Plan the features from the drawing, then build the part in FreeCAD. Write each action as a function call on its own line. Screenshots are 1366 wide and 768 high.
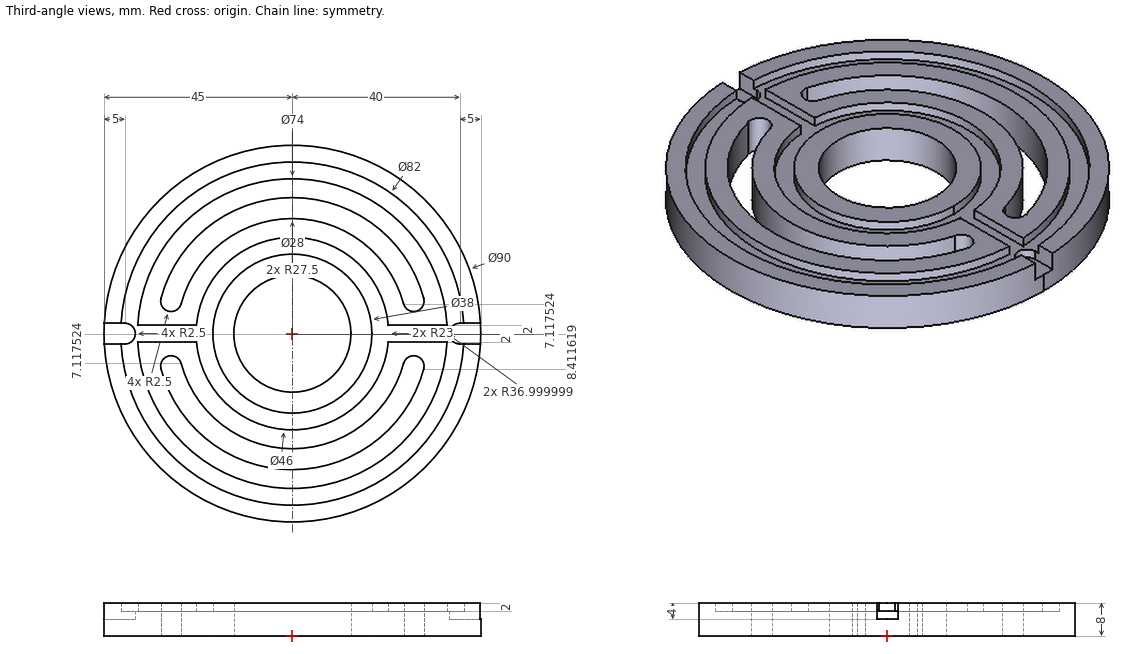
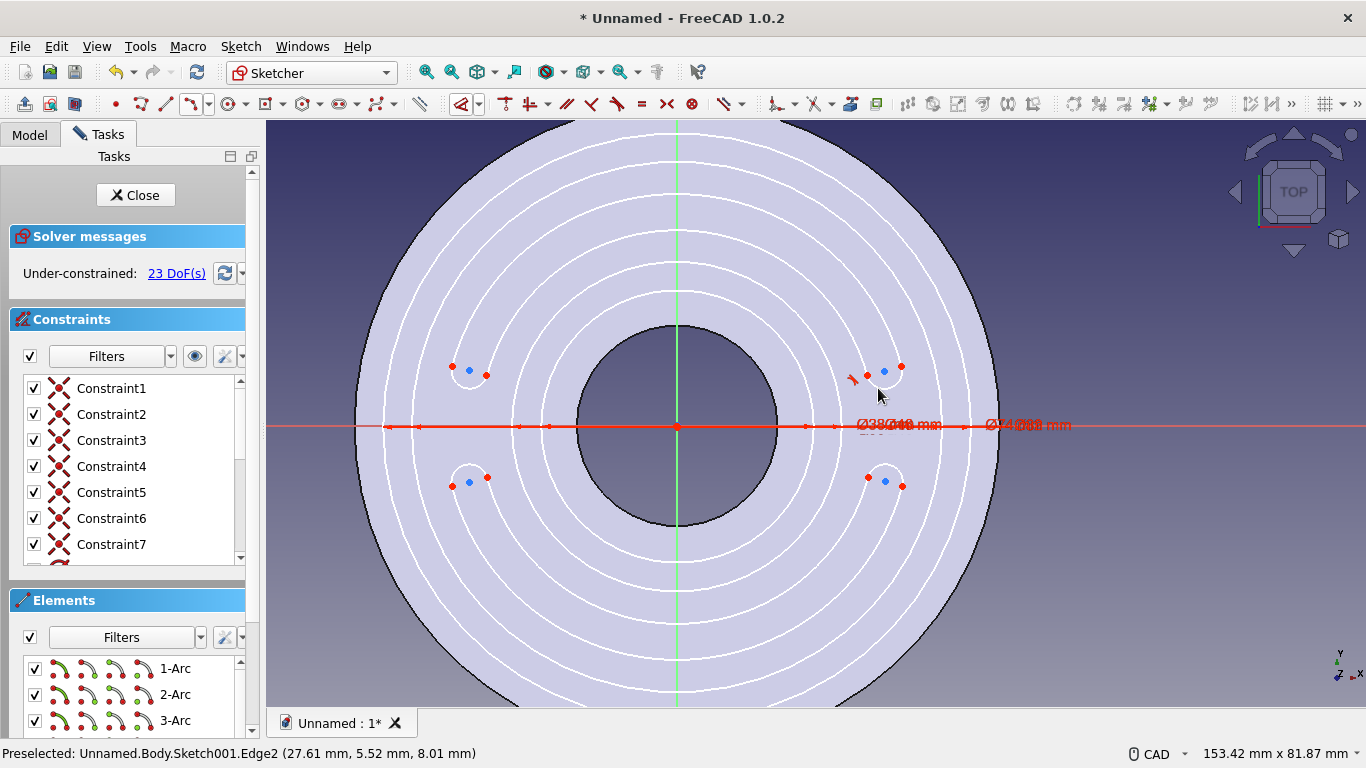
click(775, 257)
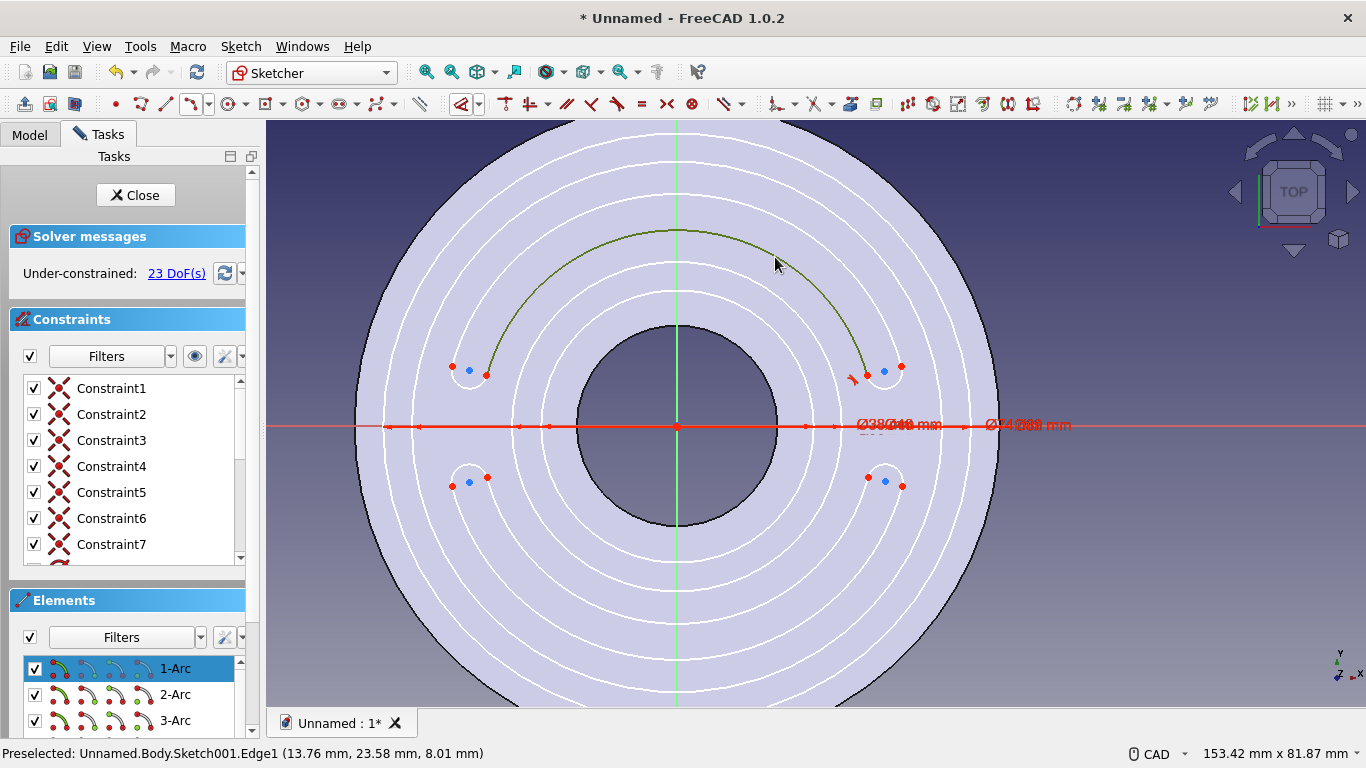
click(456, 382)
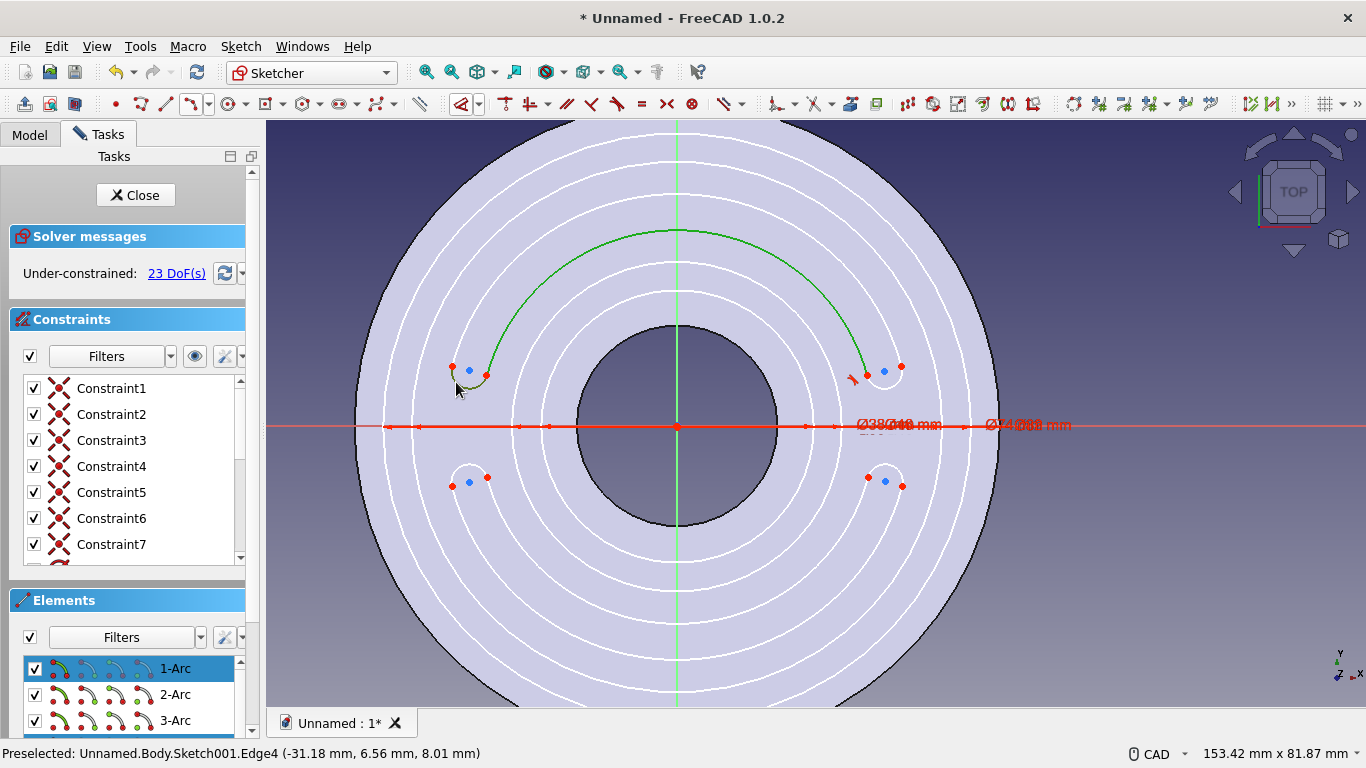
click(617, 104)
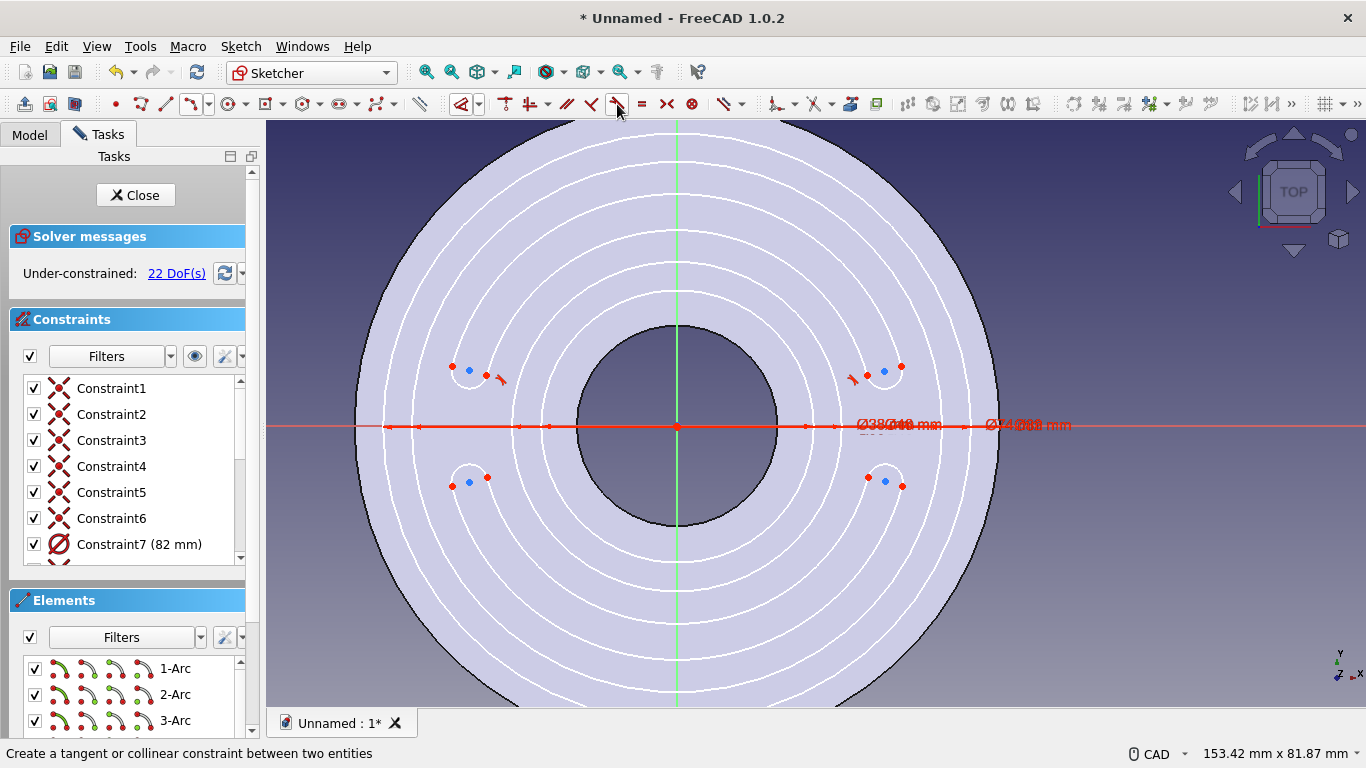
click(878, 388)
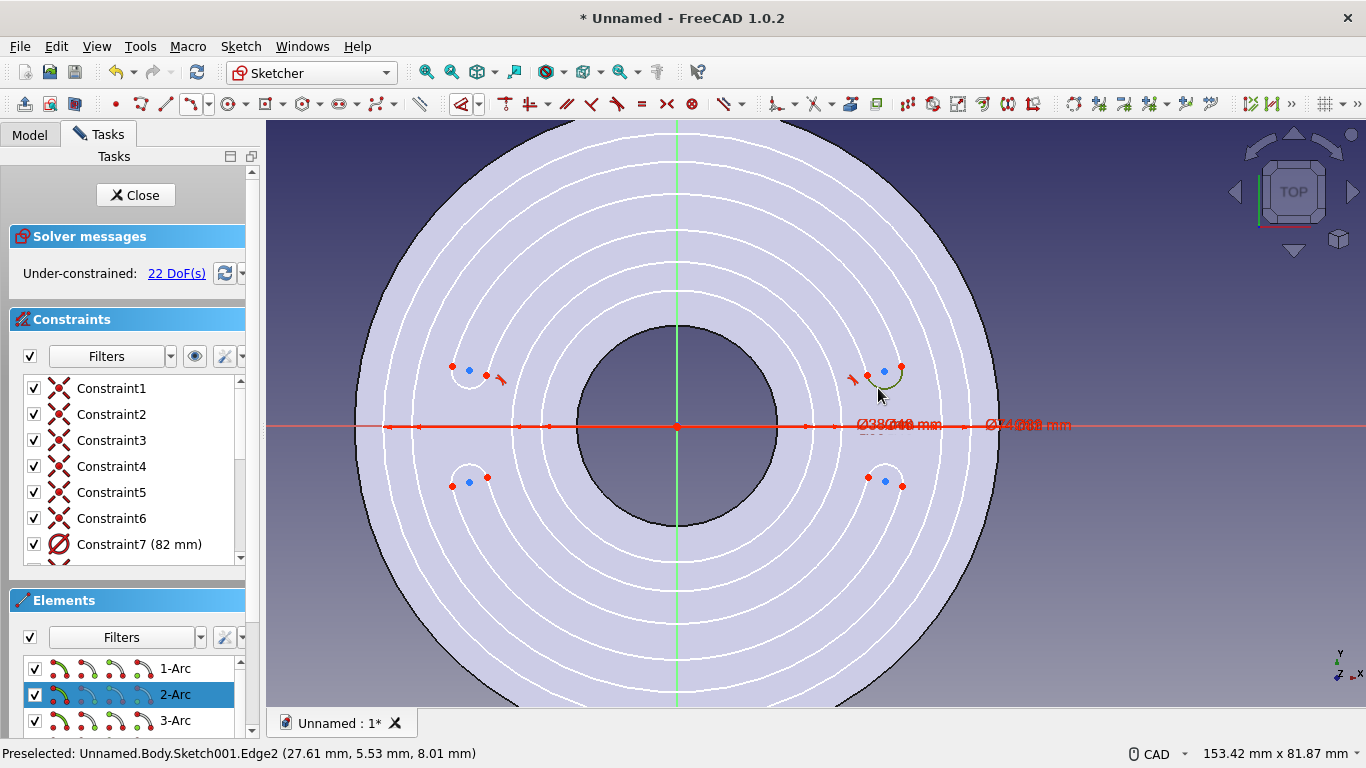
click(793, 225)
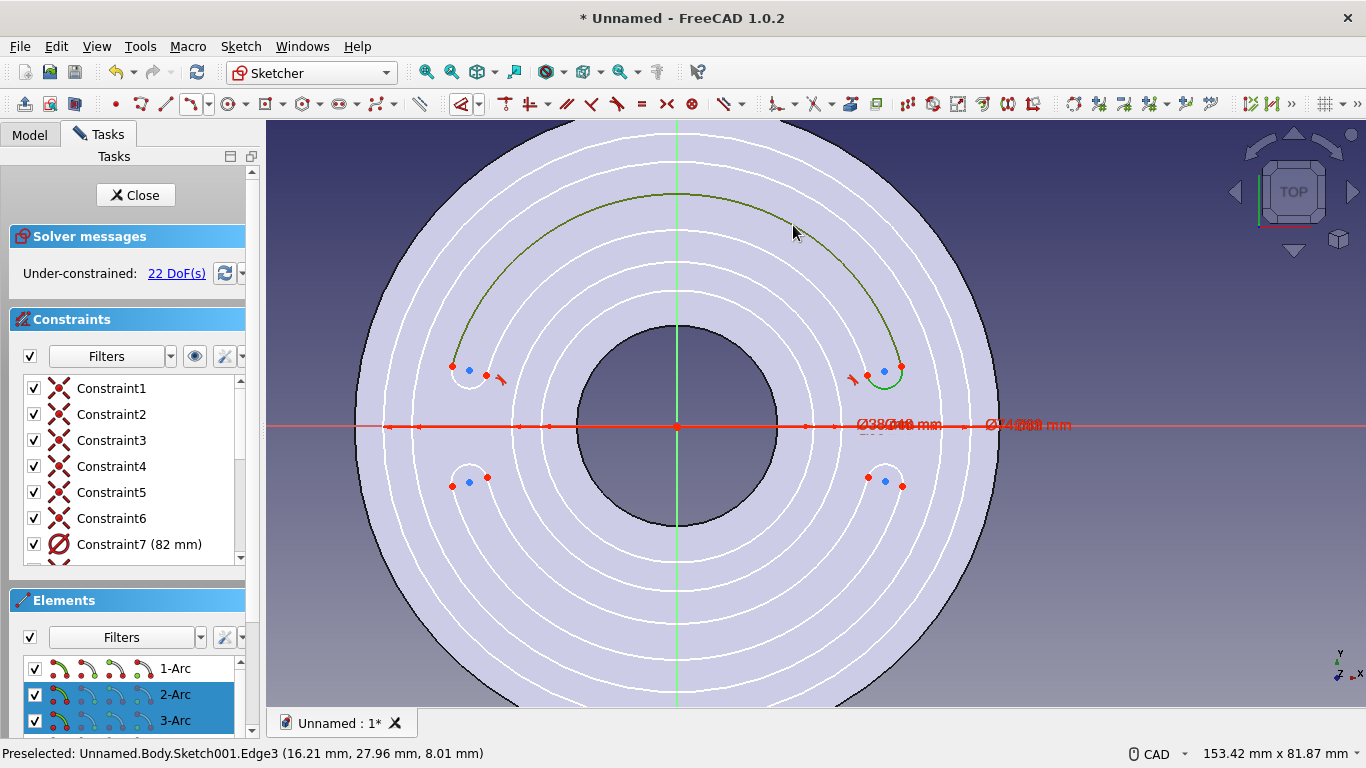
key(t)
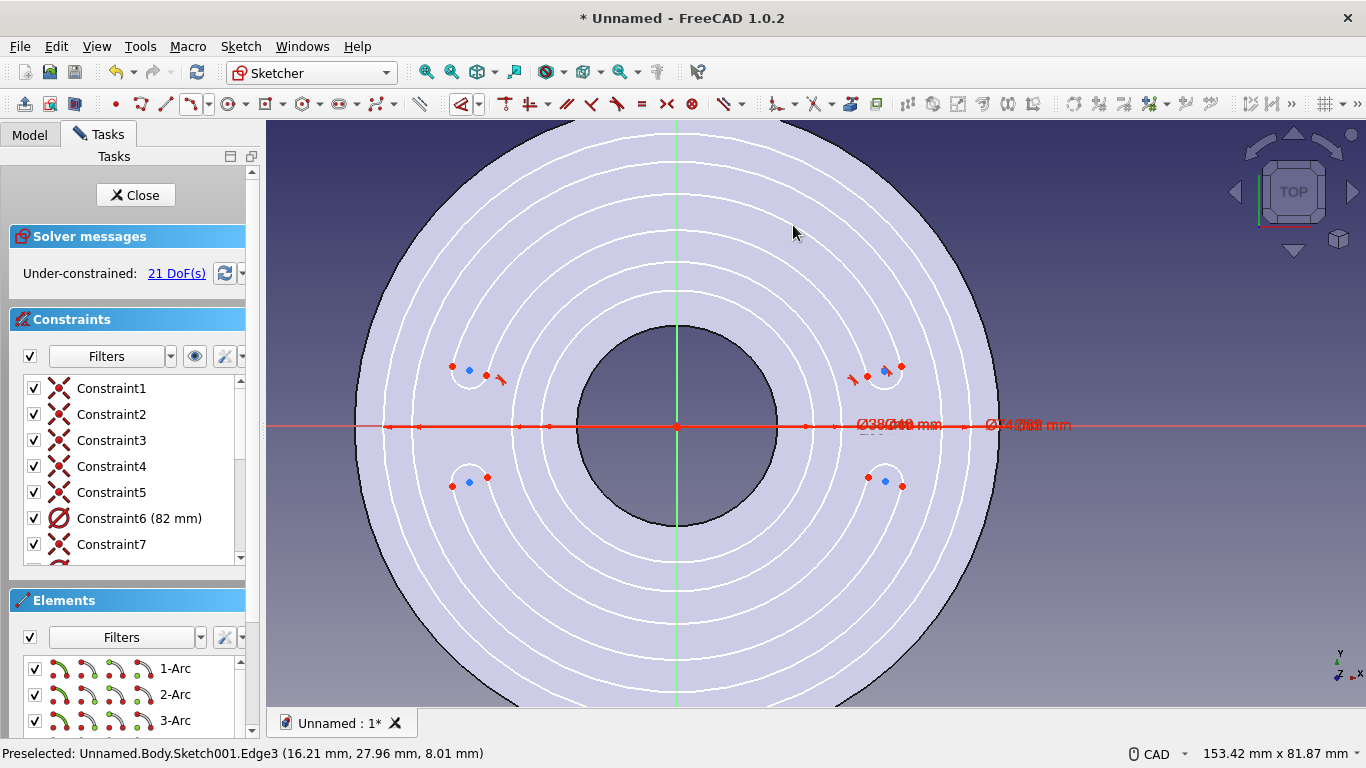
click(793, 225)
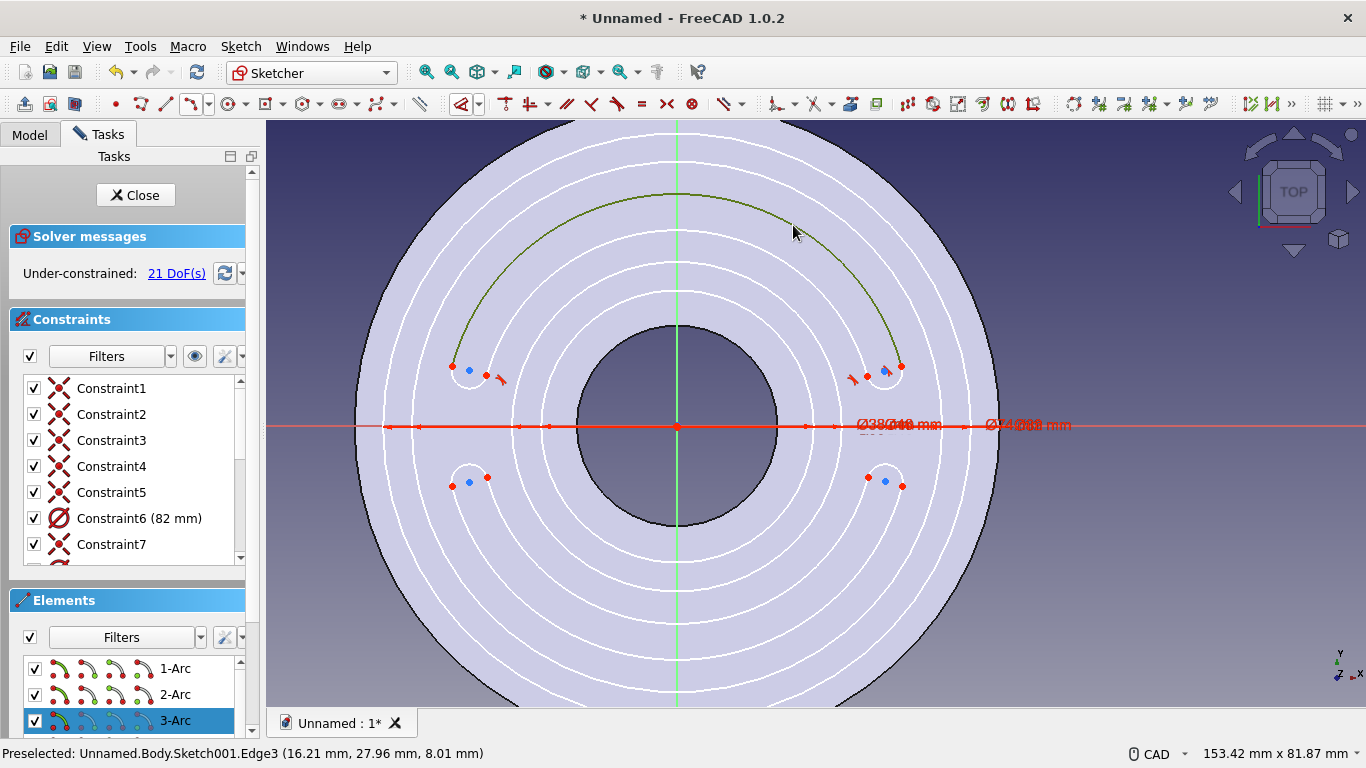
click(456, 382)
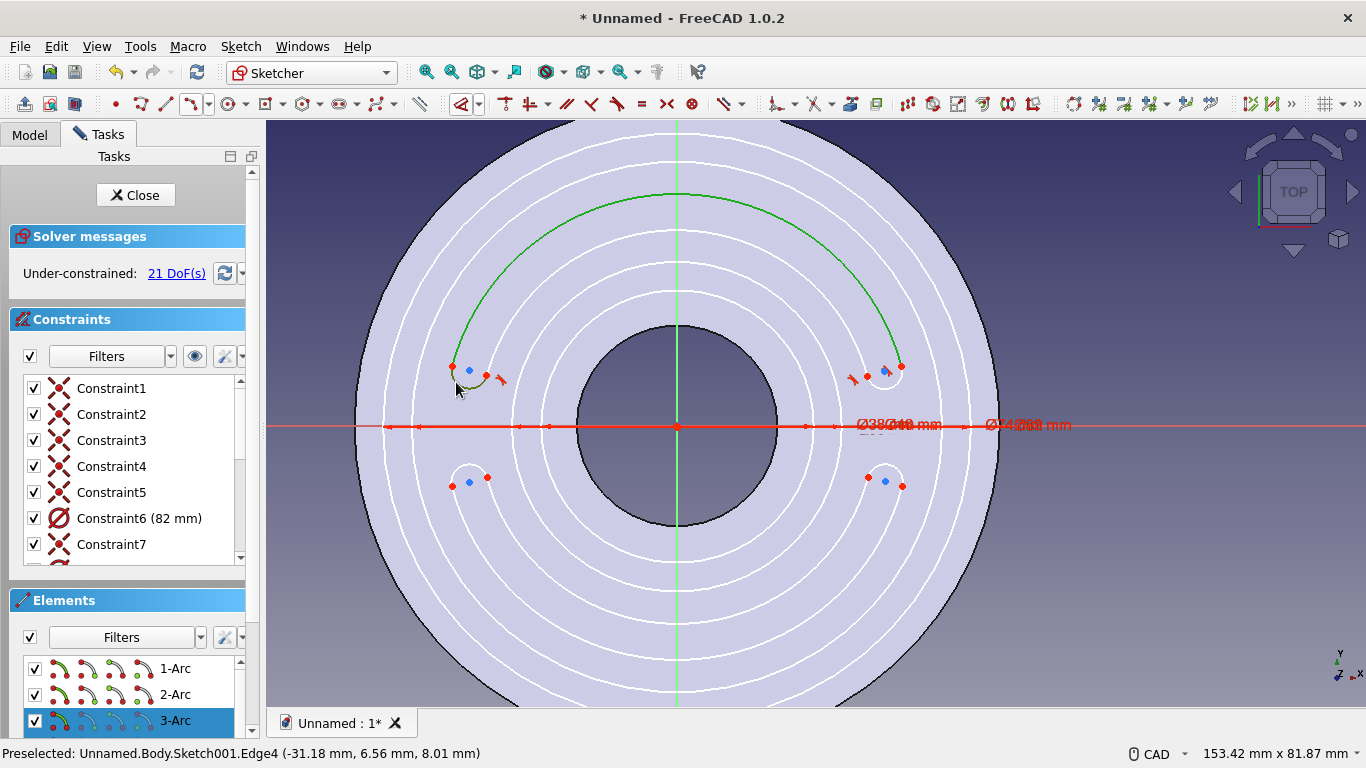
click(617, 104)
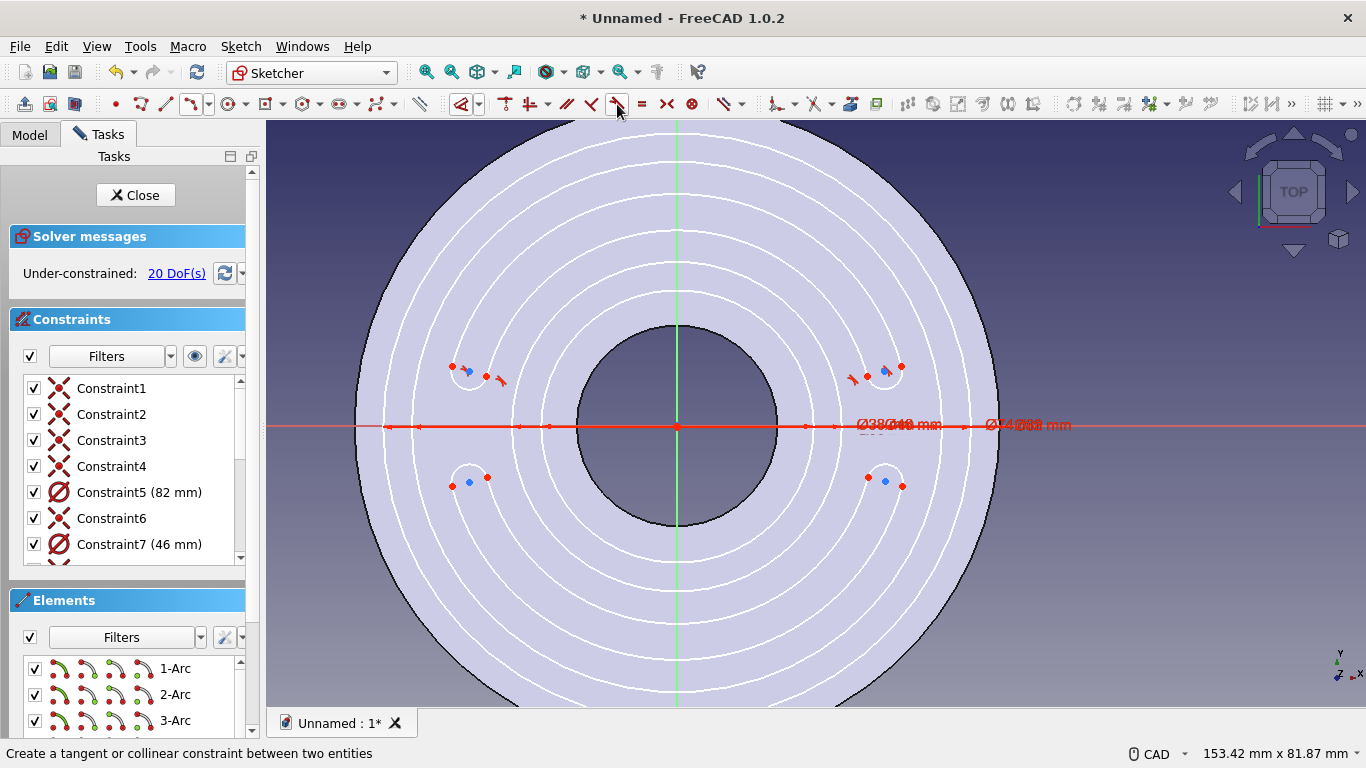
click(476, 466)